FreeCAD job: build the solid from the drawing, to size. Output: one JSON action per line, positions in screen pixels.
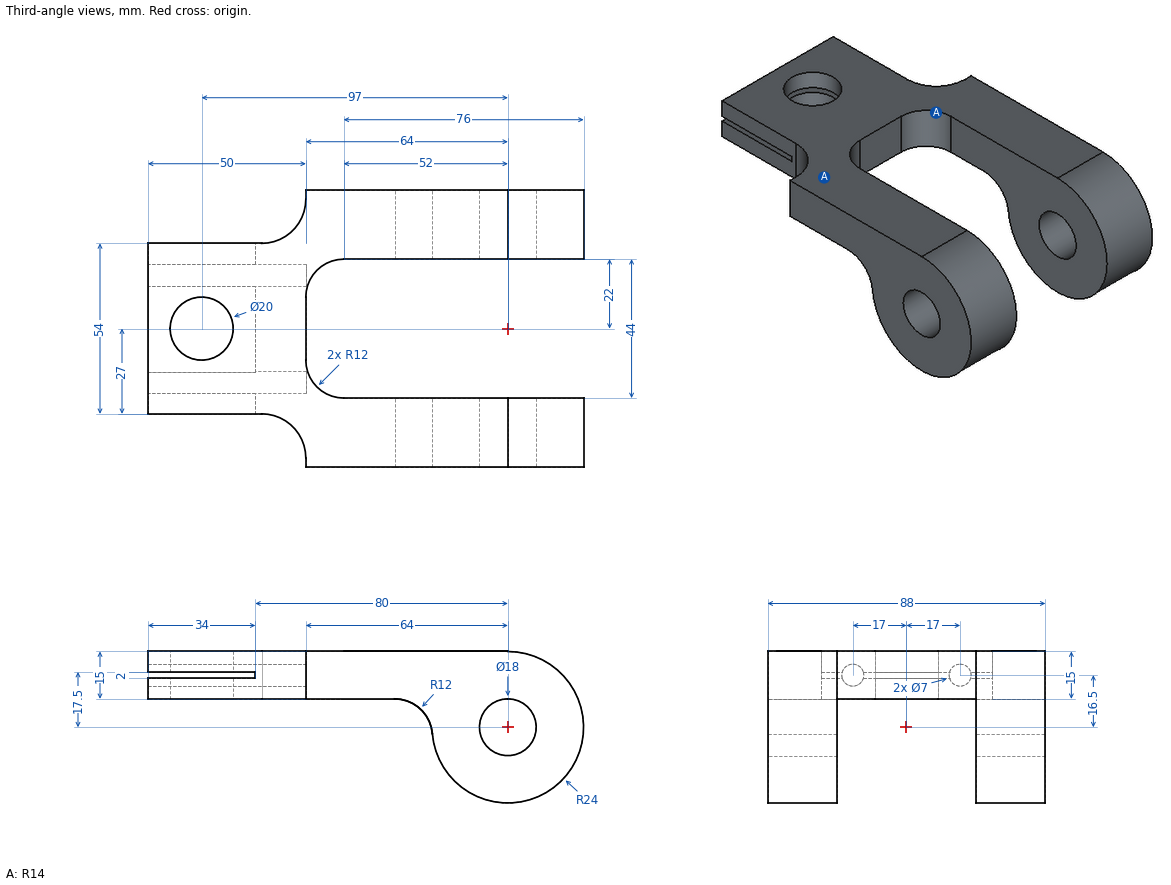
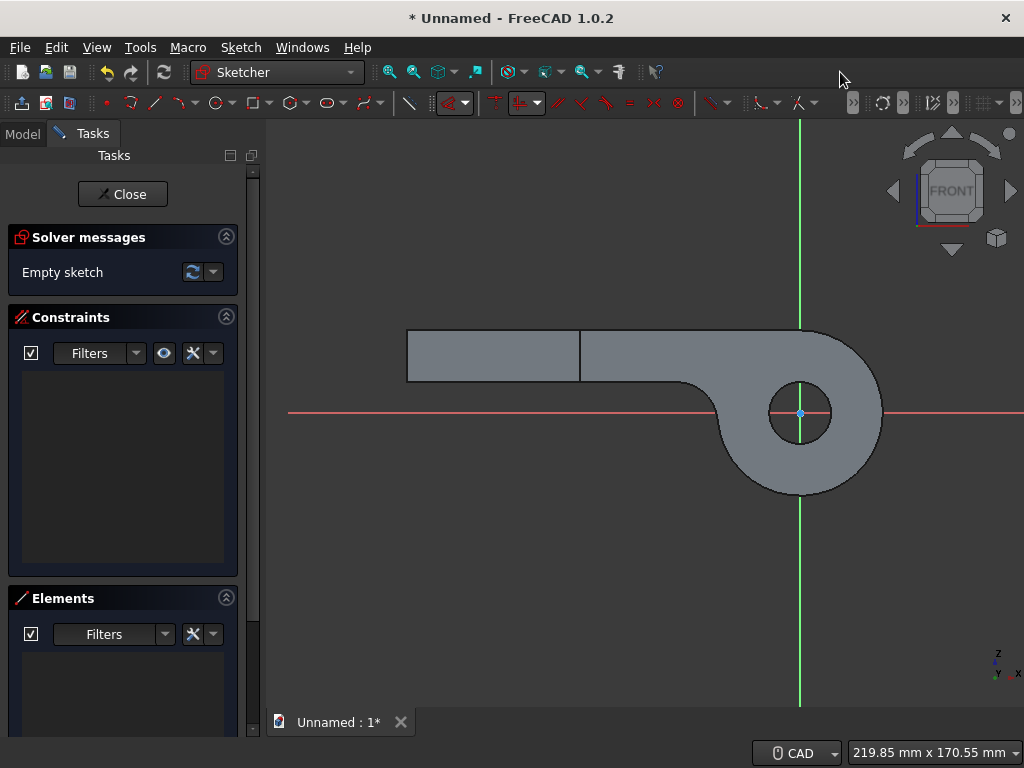
{"action": "scroll", "coordinate": [418, 332], "scroll_direction": "up", "scroll_amount": 6}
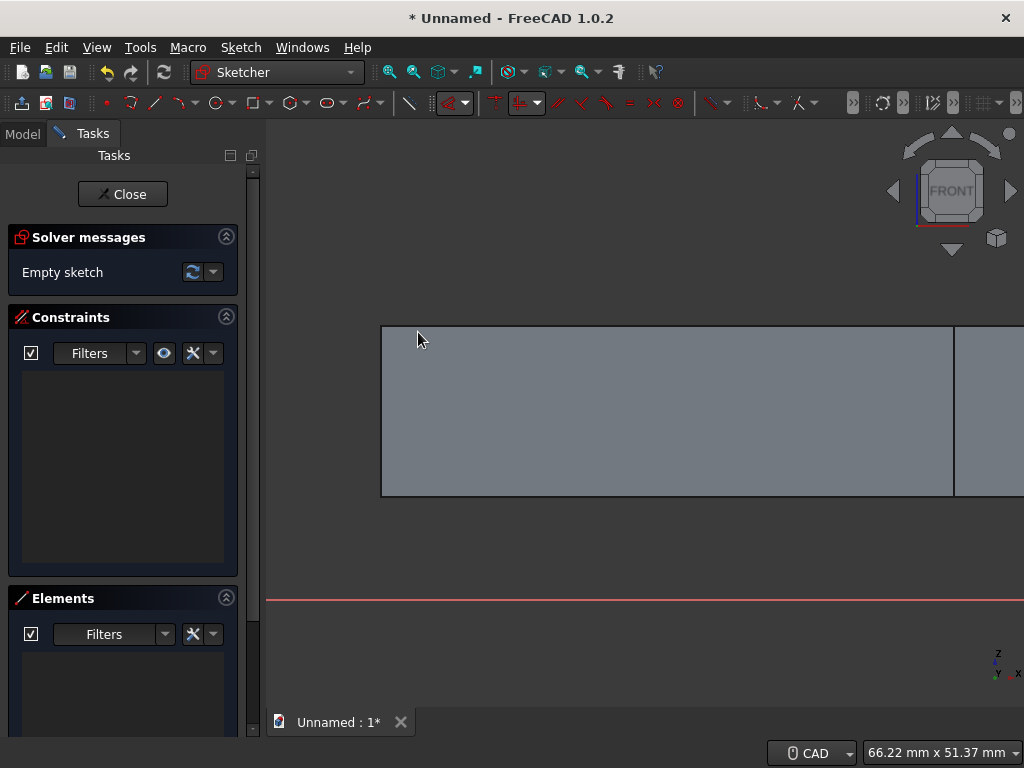
{"action": "left_click", "coordinate": [254, 104]}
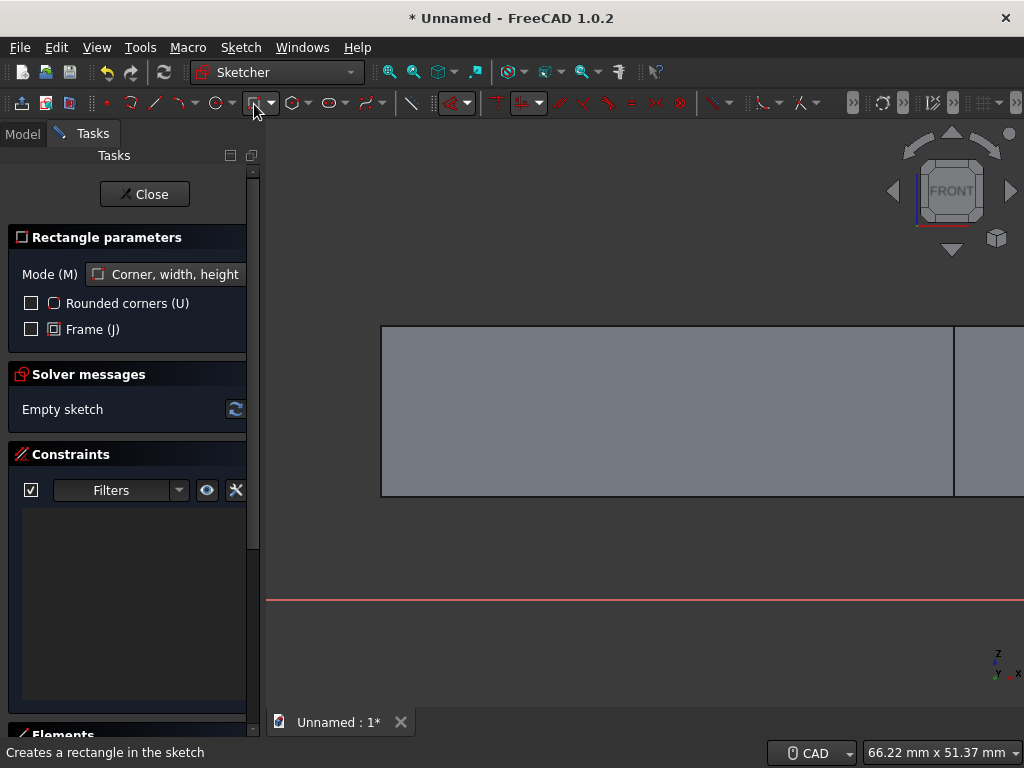
{"action": "left_click", "coordinate": [381, 400]}
{"action": "left_click", "coordinate": [771, 423]}
{"action": "key", "text": "Escape"}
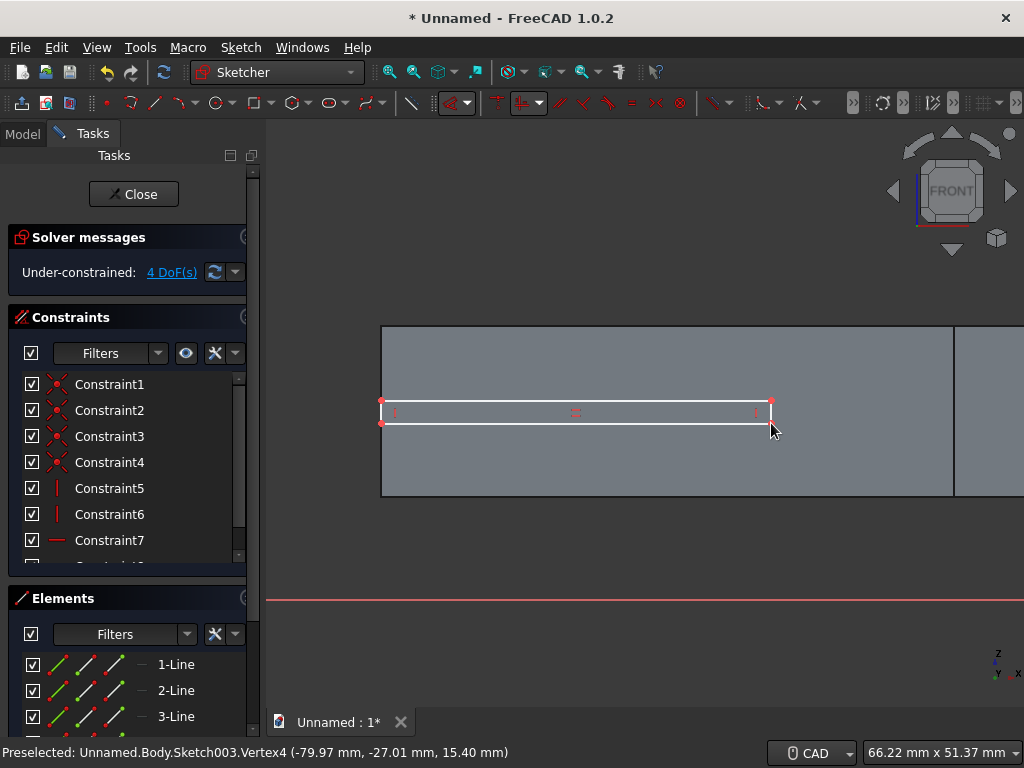
{"action": "scroll", "coordinate": [381, 410], "scroll_direction": "up", "scroll_amount": 3}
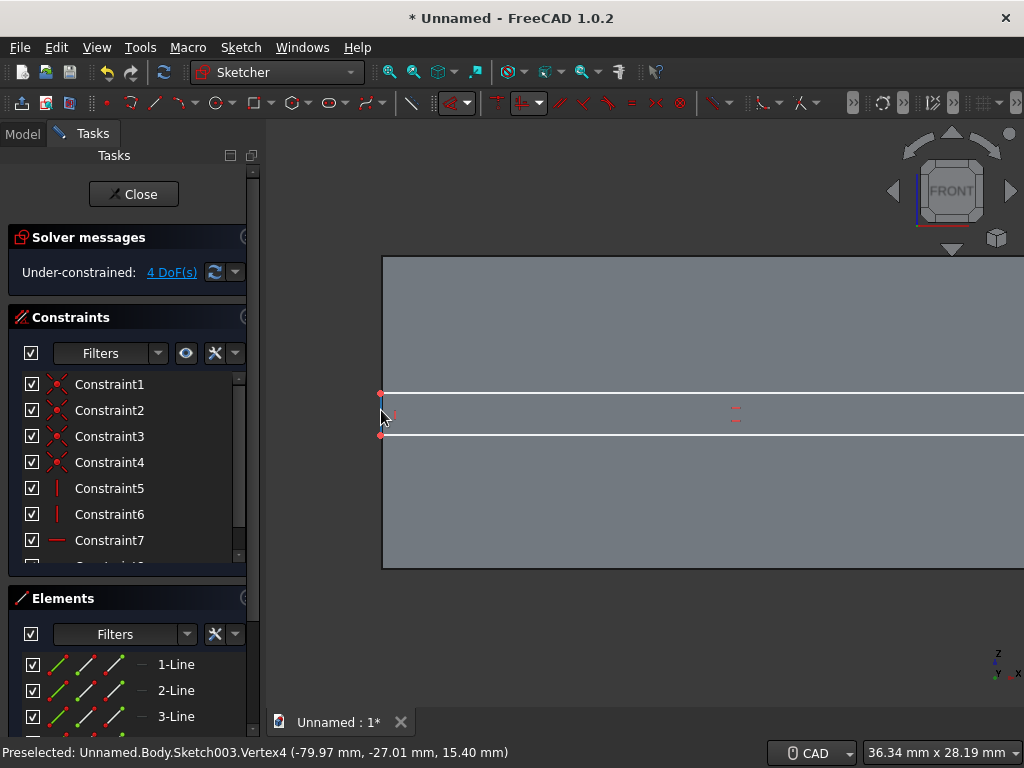
{"action": "left_click", "coordinate": [381, 410]}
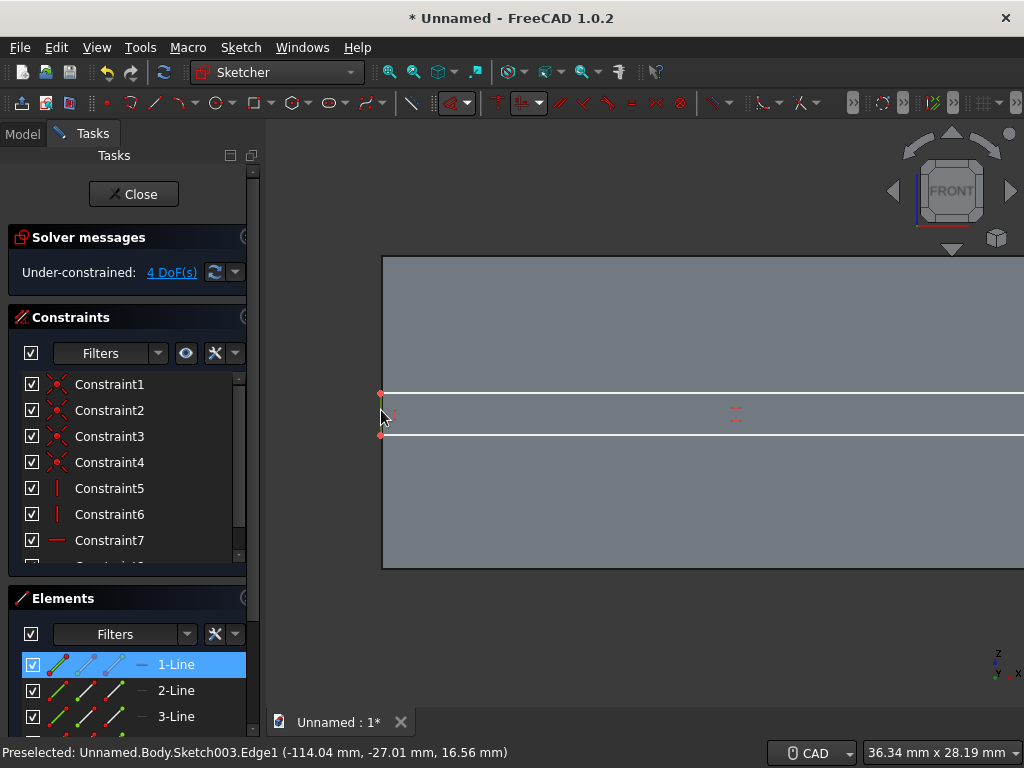
{"action": "key", "text": "i"}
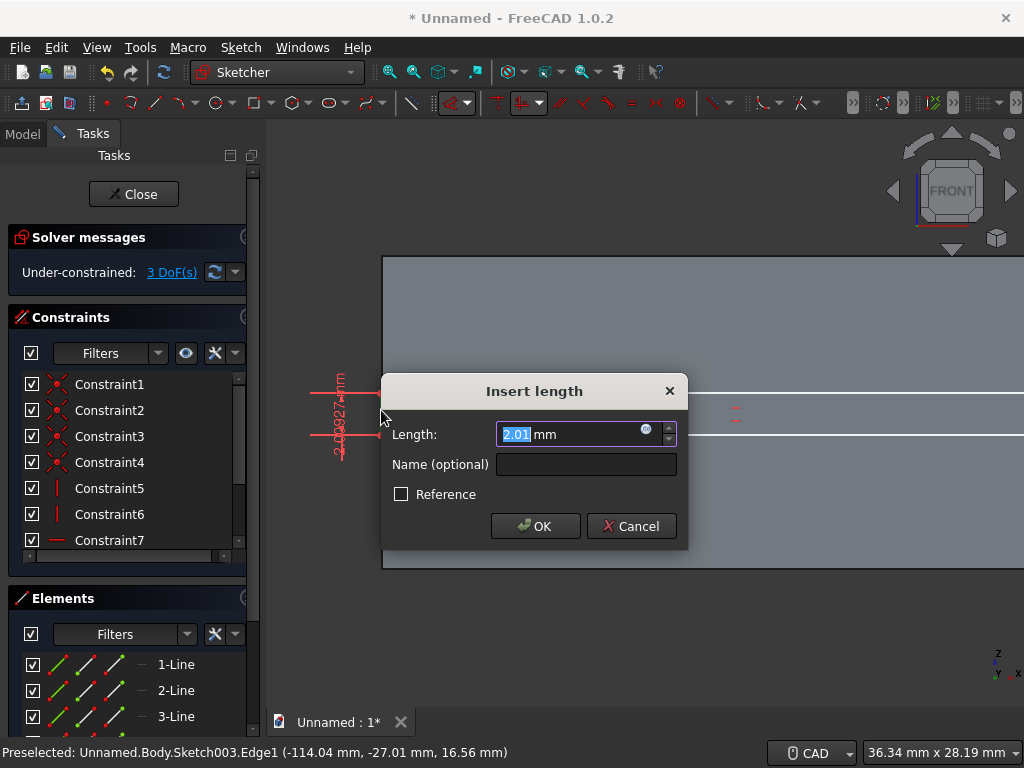
{"action": "type", "text": "2"}
{"action": "key", "text": "Return"}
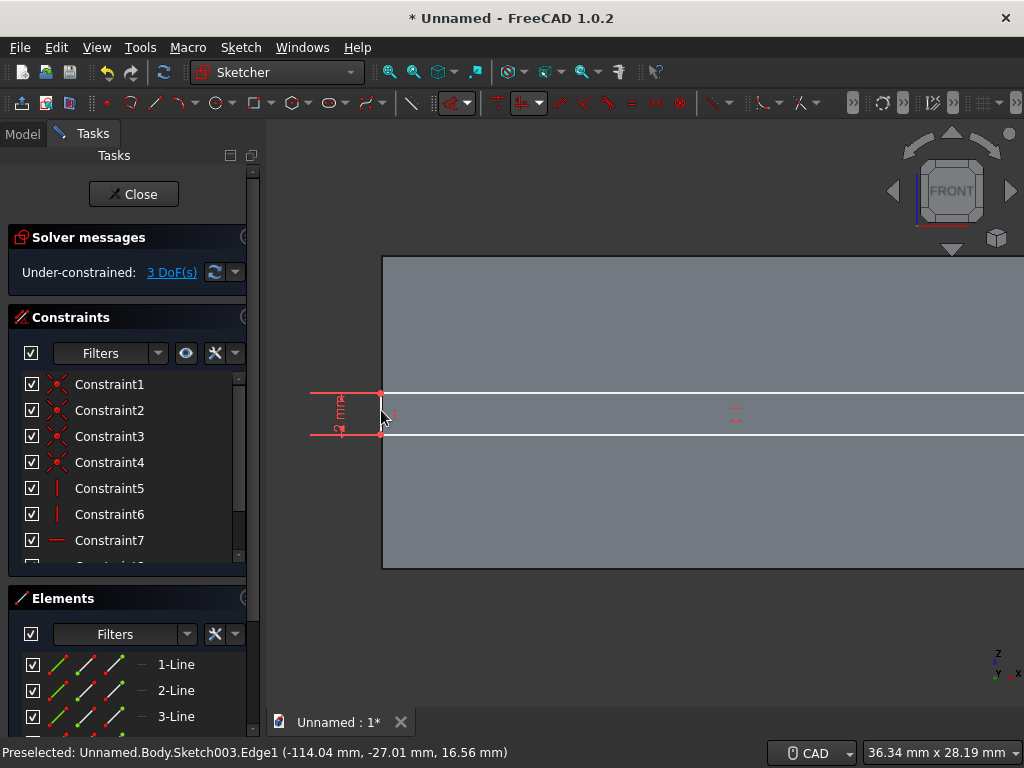
{"action": "left_click", "coordinate": [594, 435]}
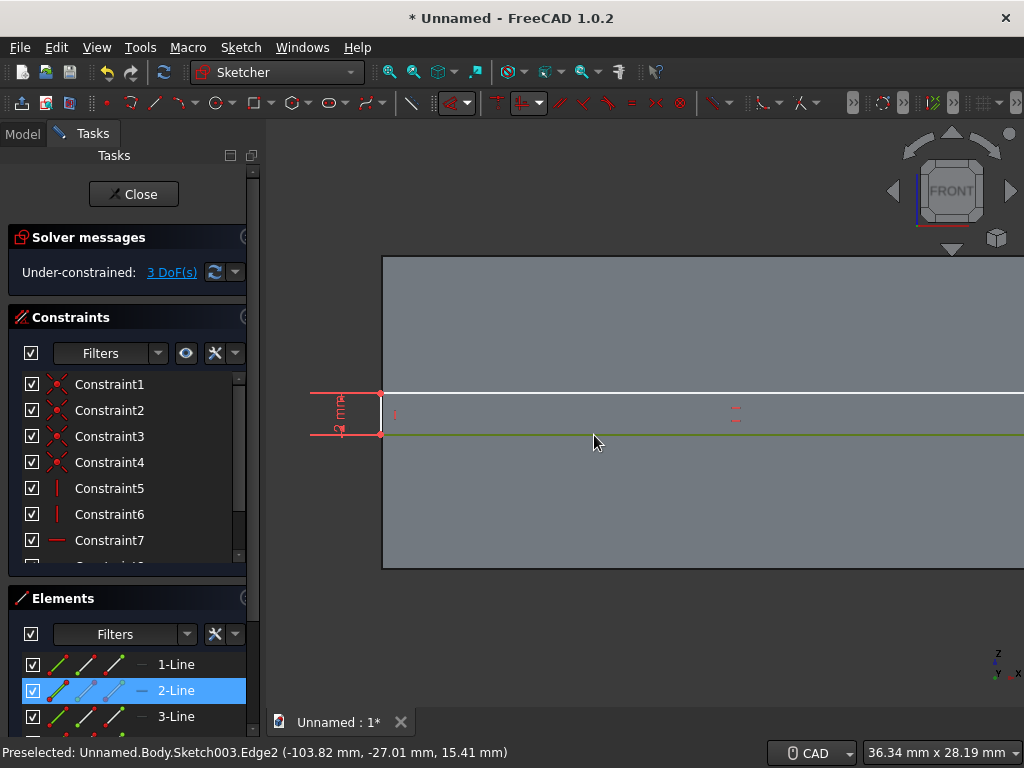
{"action": "left_click", "coordinate": [470, 104]}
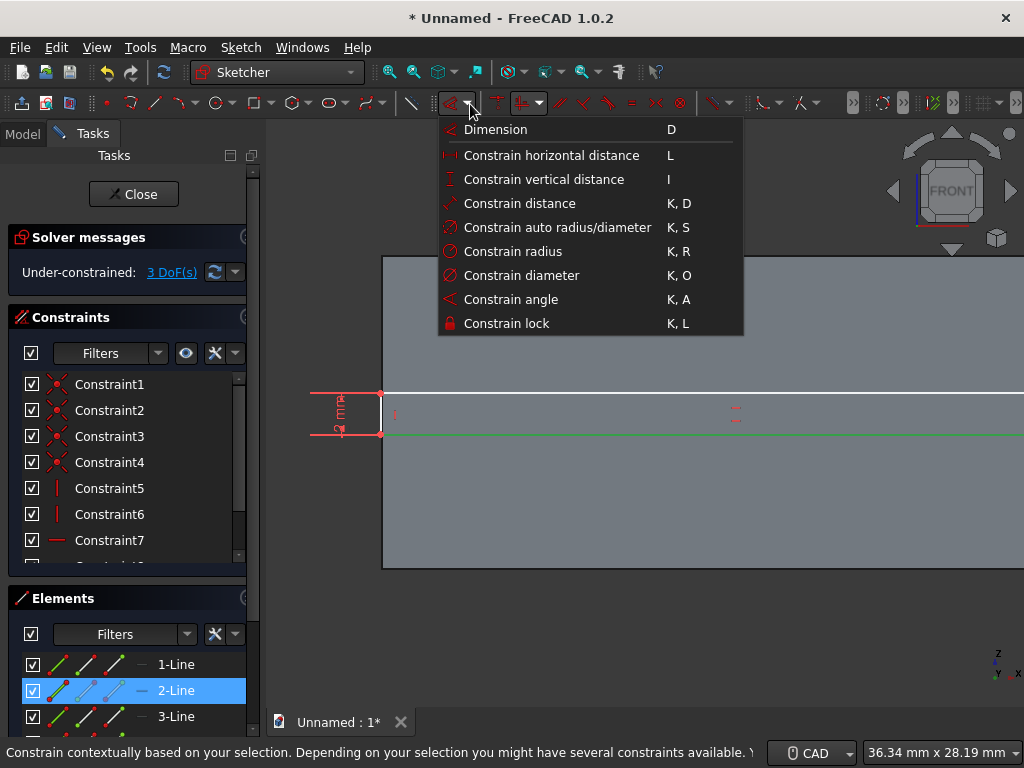
{"action": "left_click", "coordinate": [591, 155]}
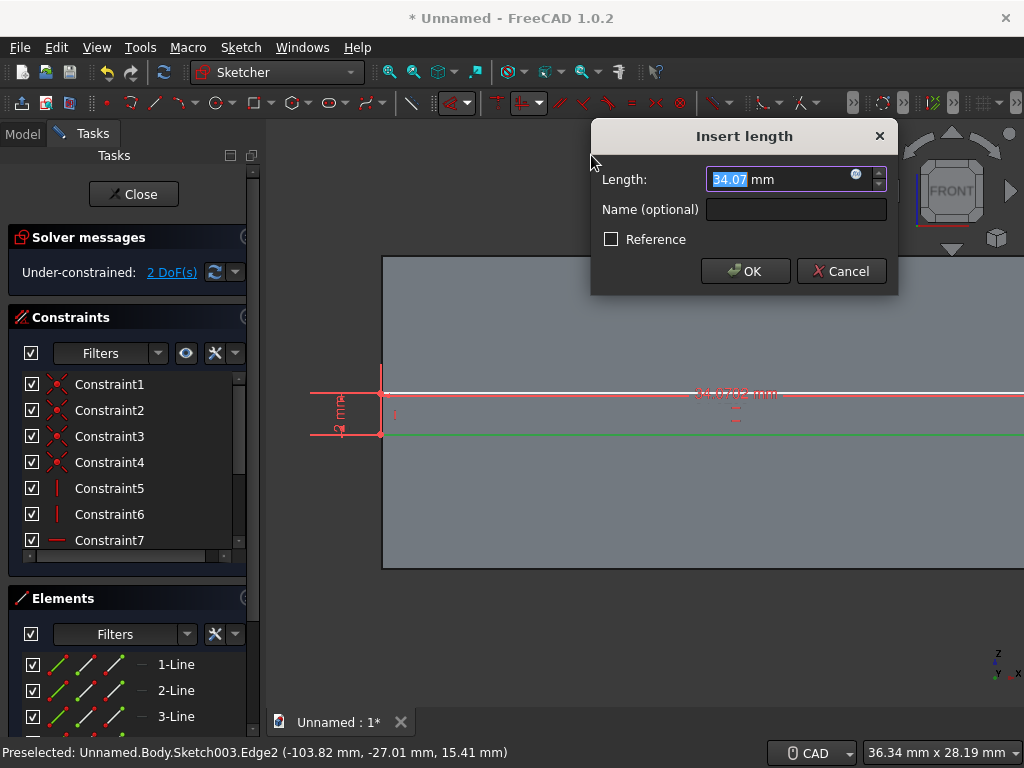
{"action": "type", "text": "34"}
{"action": "key", "text": "Return"}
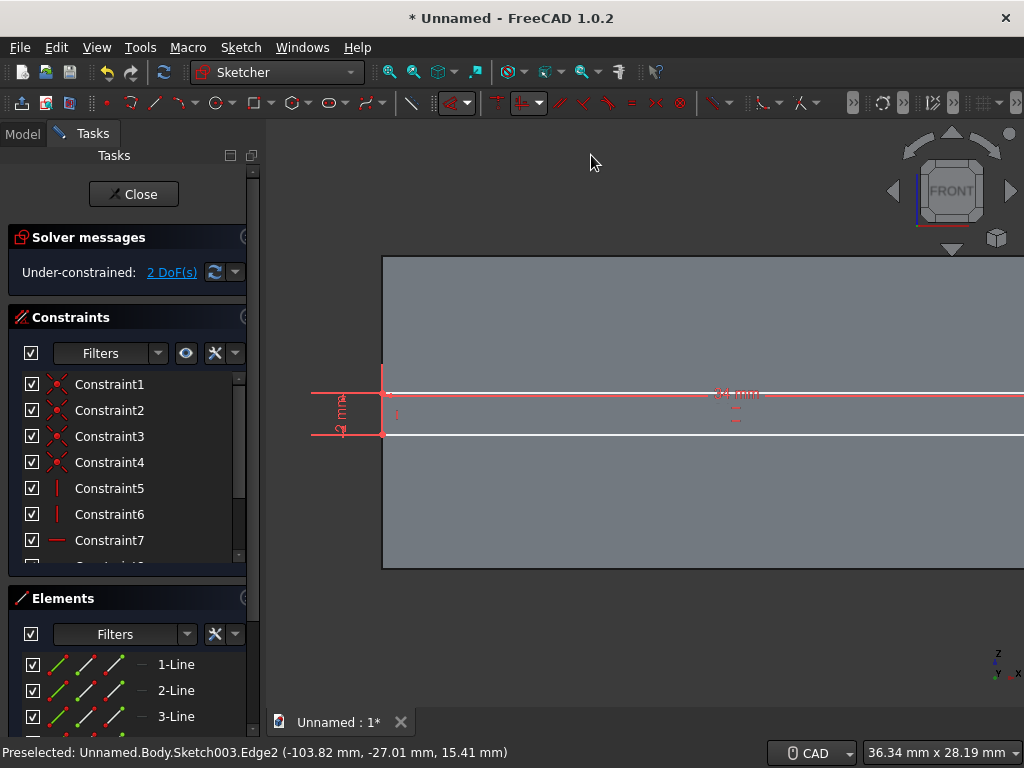
{"action": "scroll", "coordinate": [382, 414], "scroll_direction": "down", "scroll_amount": 3}